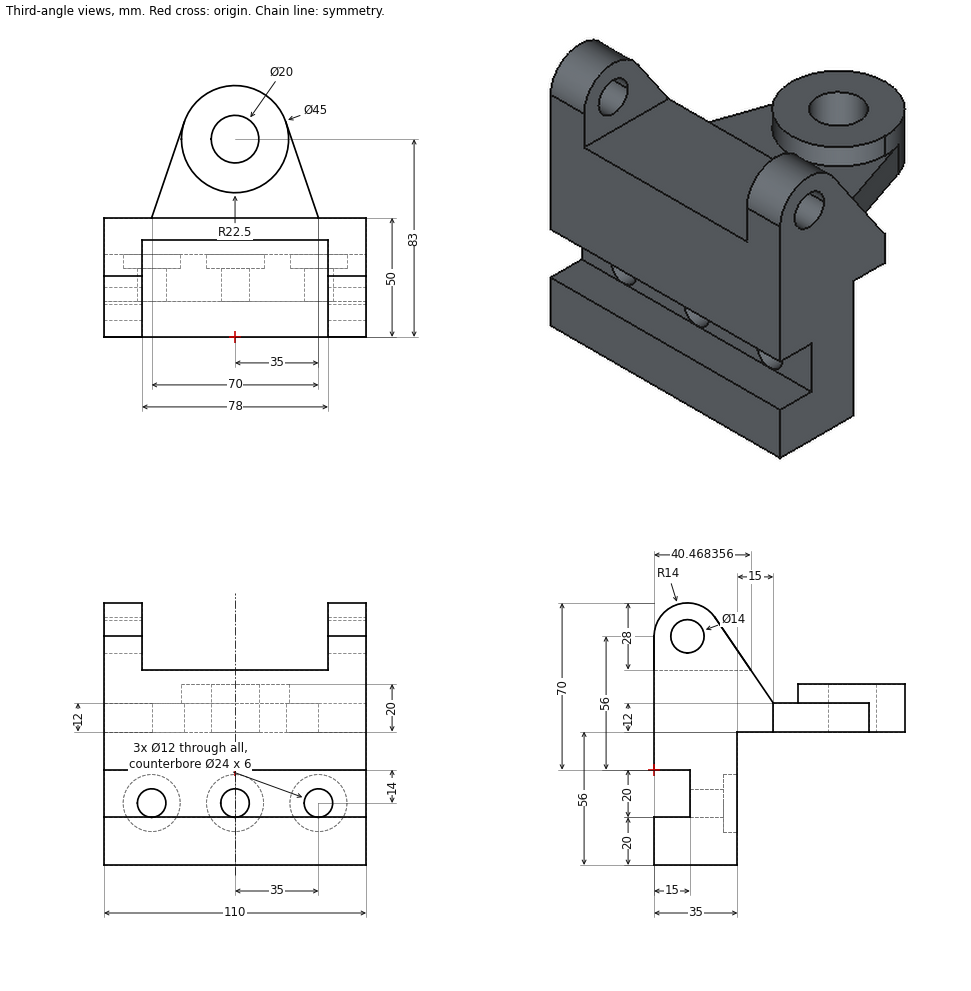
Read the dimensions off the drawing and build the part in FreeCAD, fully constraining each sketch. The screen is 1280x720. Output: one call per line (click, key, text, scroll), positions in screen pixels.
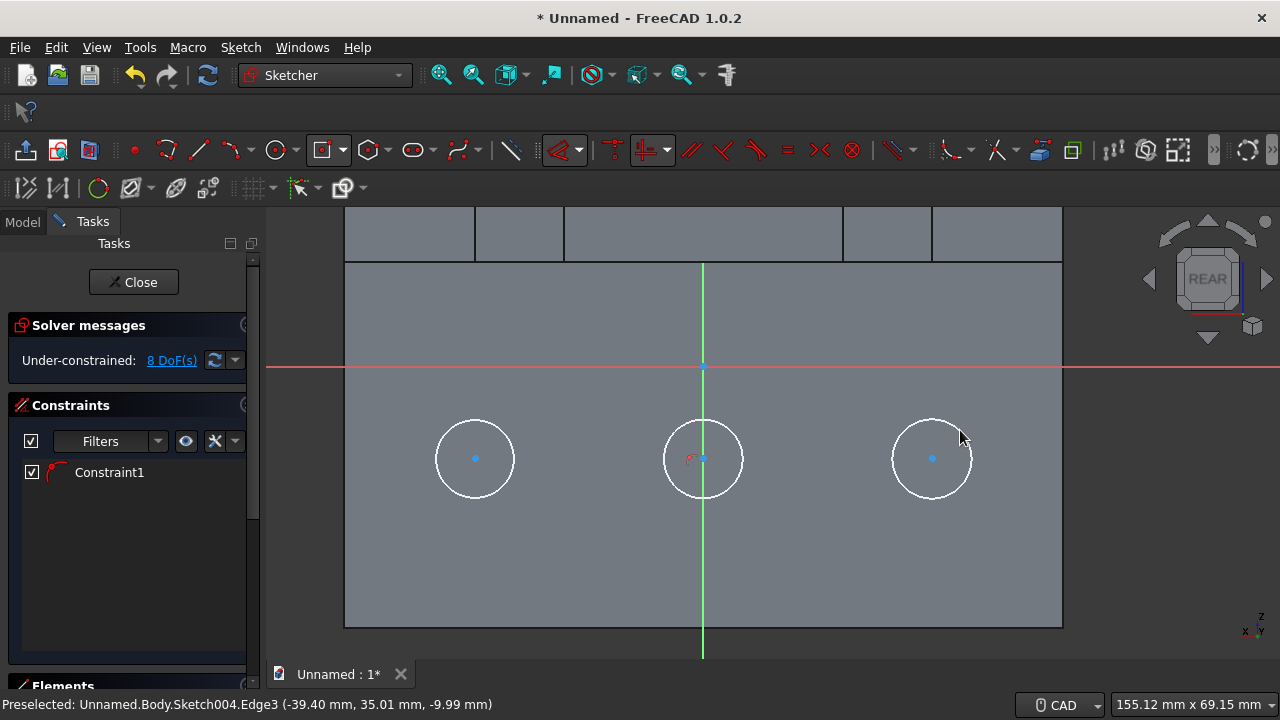
click(502, 431)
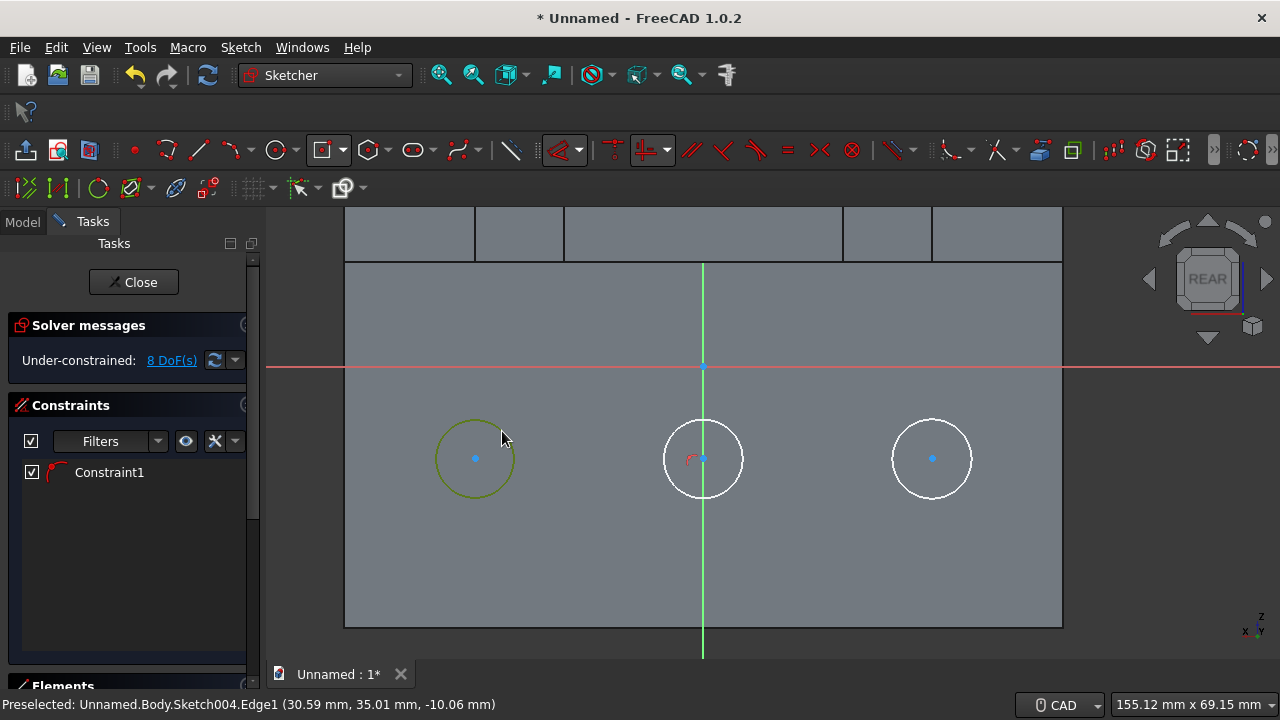
click(731, 431)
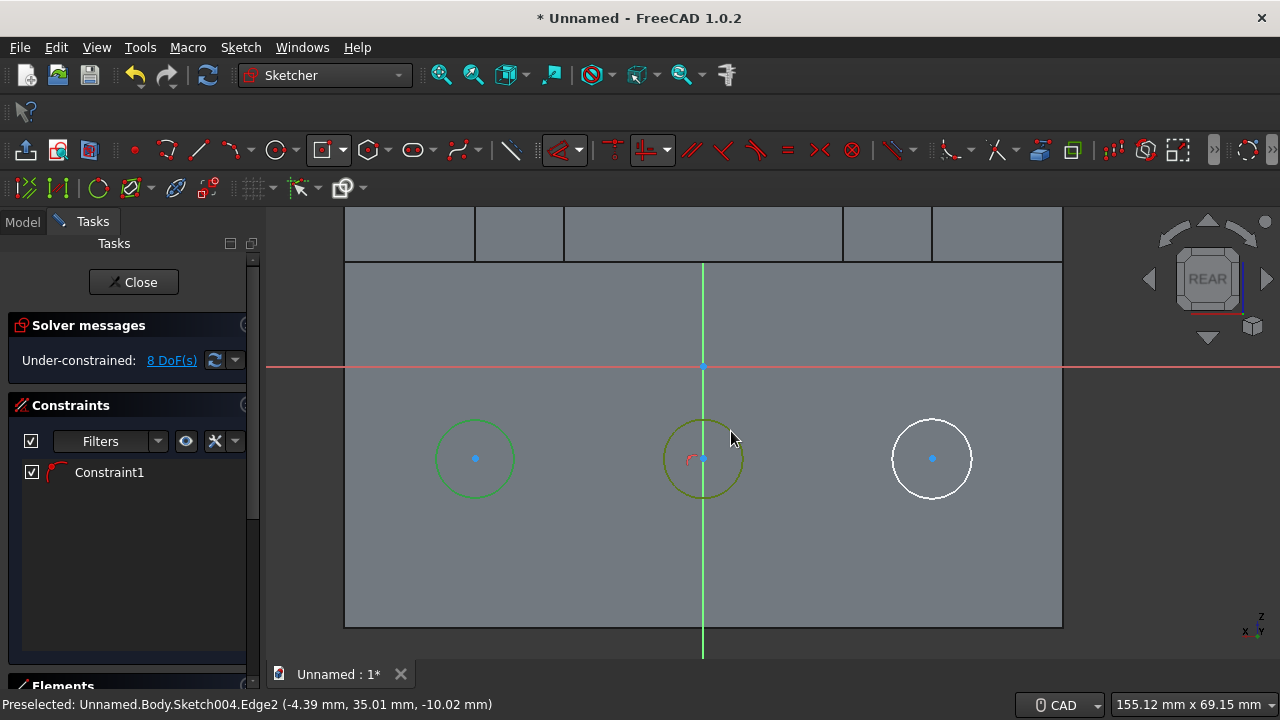
click(960, 431)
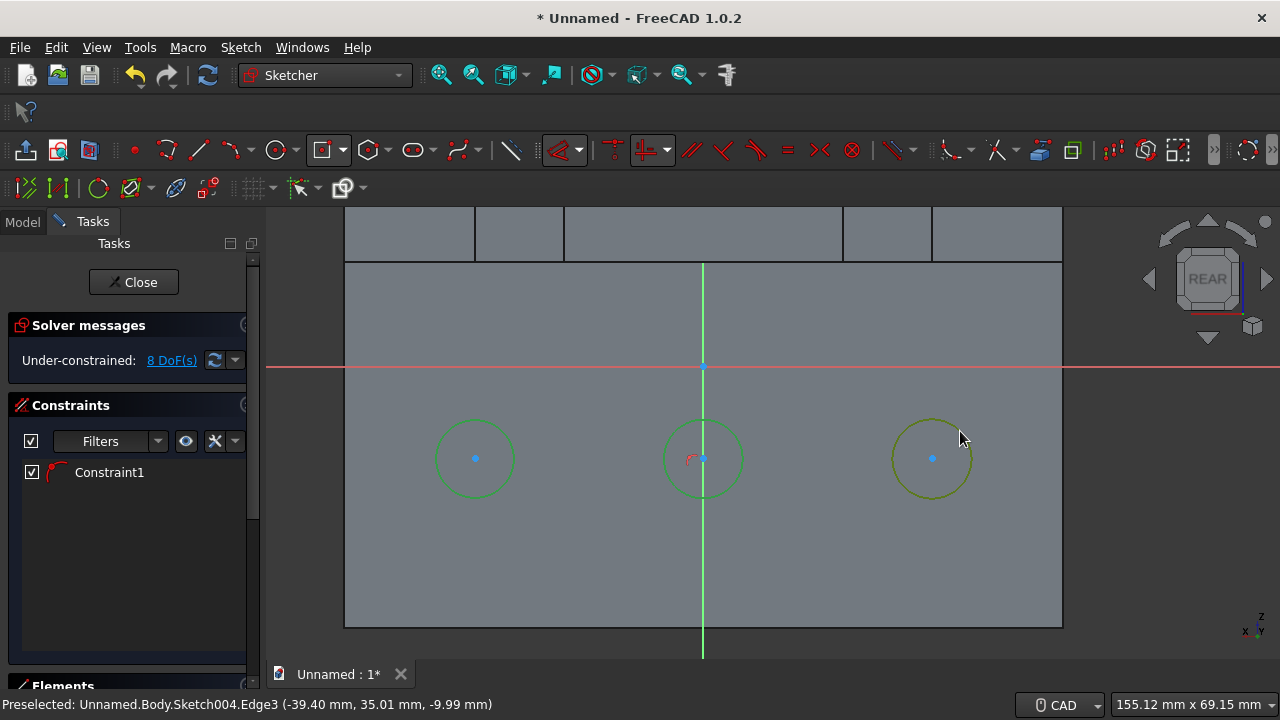
click(788, 150)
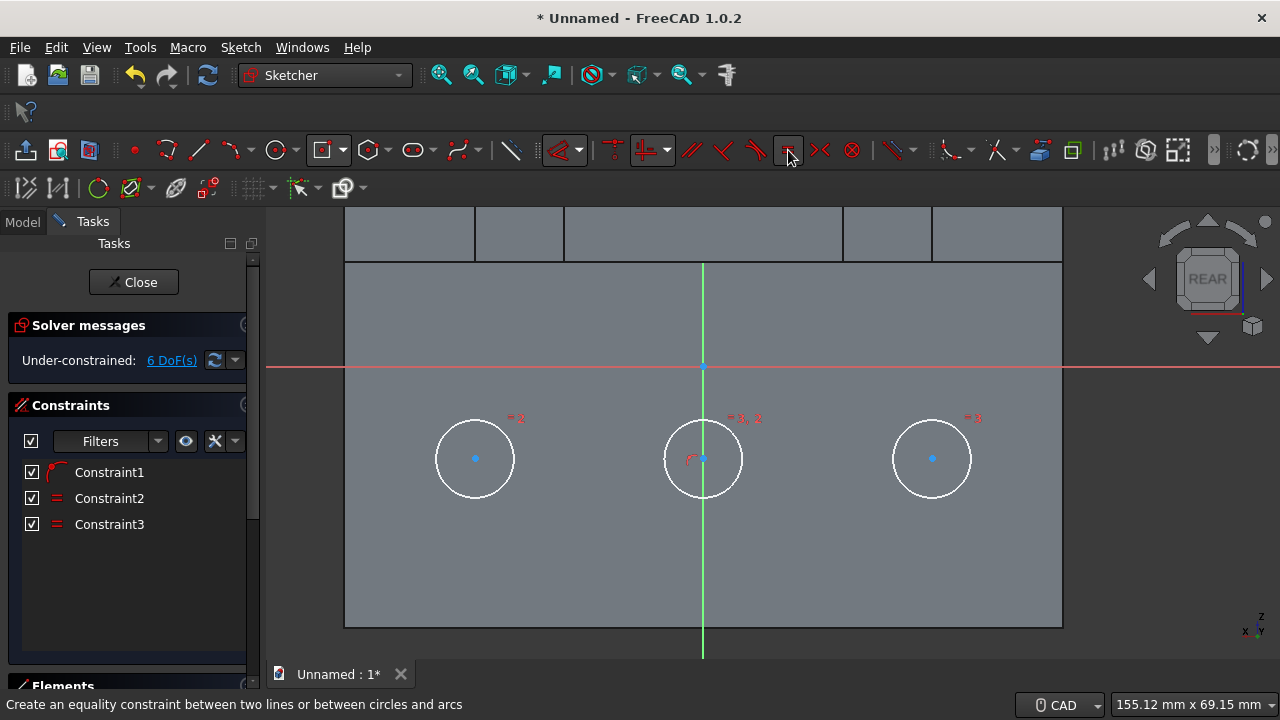
click(475, 459)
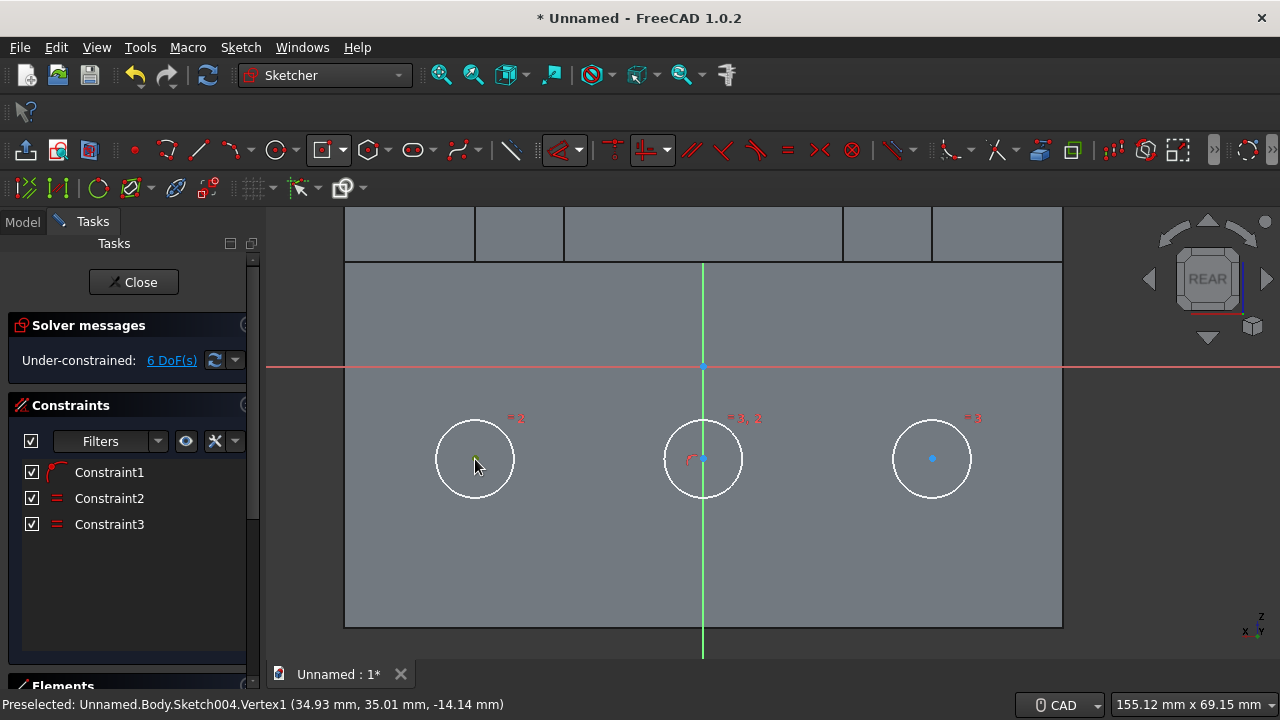
click(932, 459)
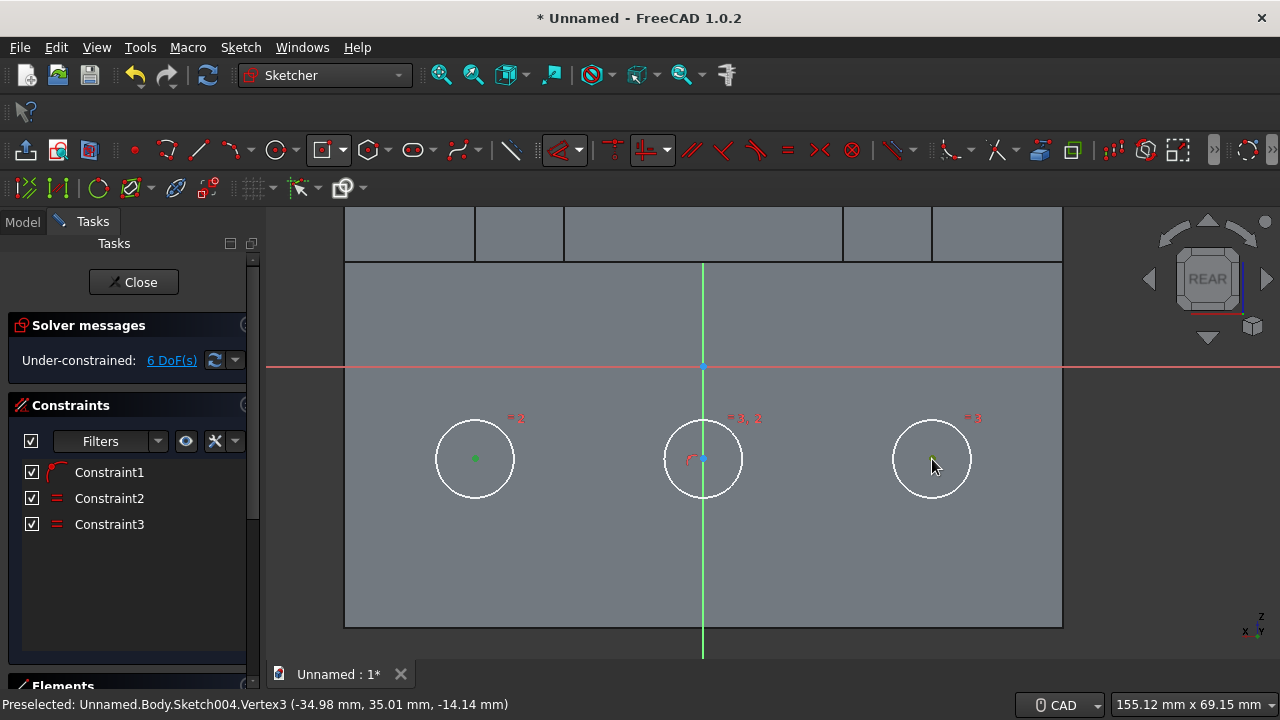
click(703, 603)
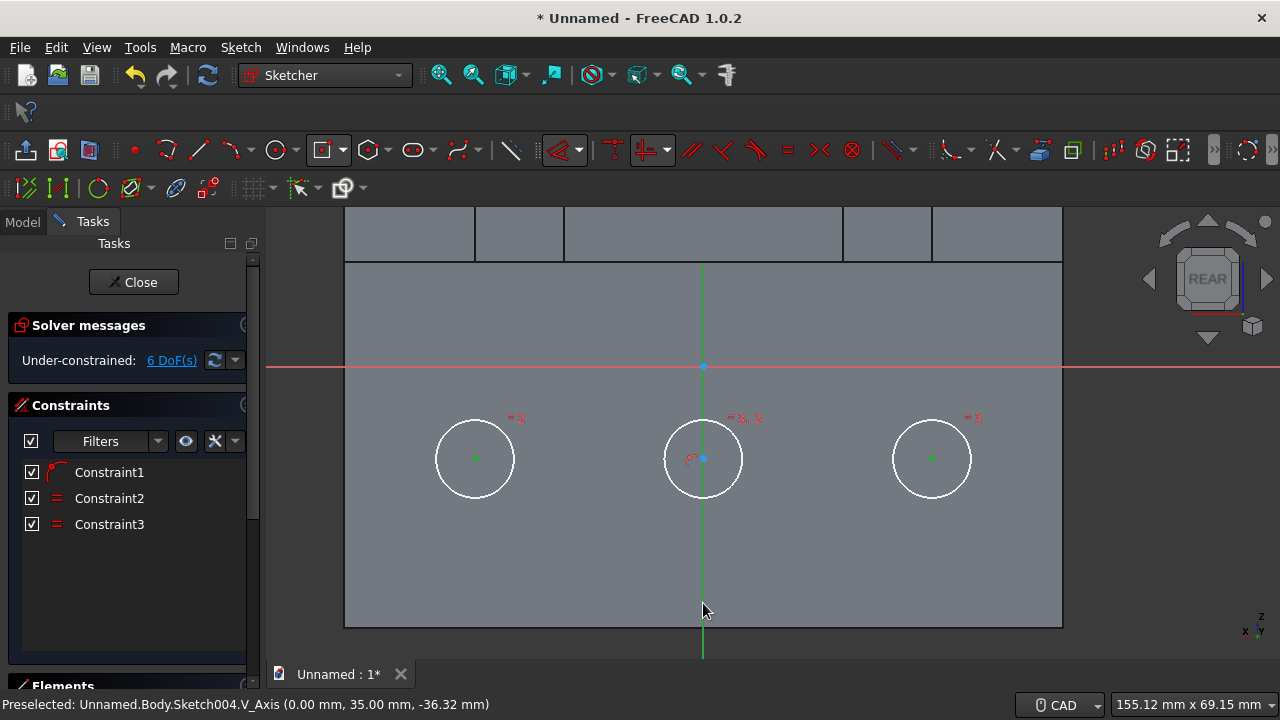
click(820, 150)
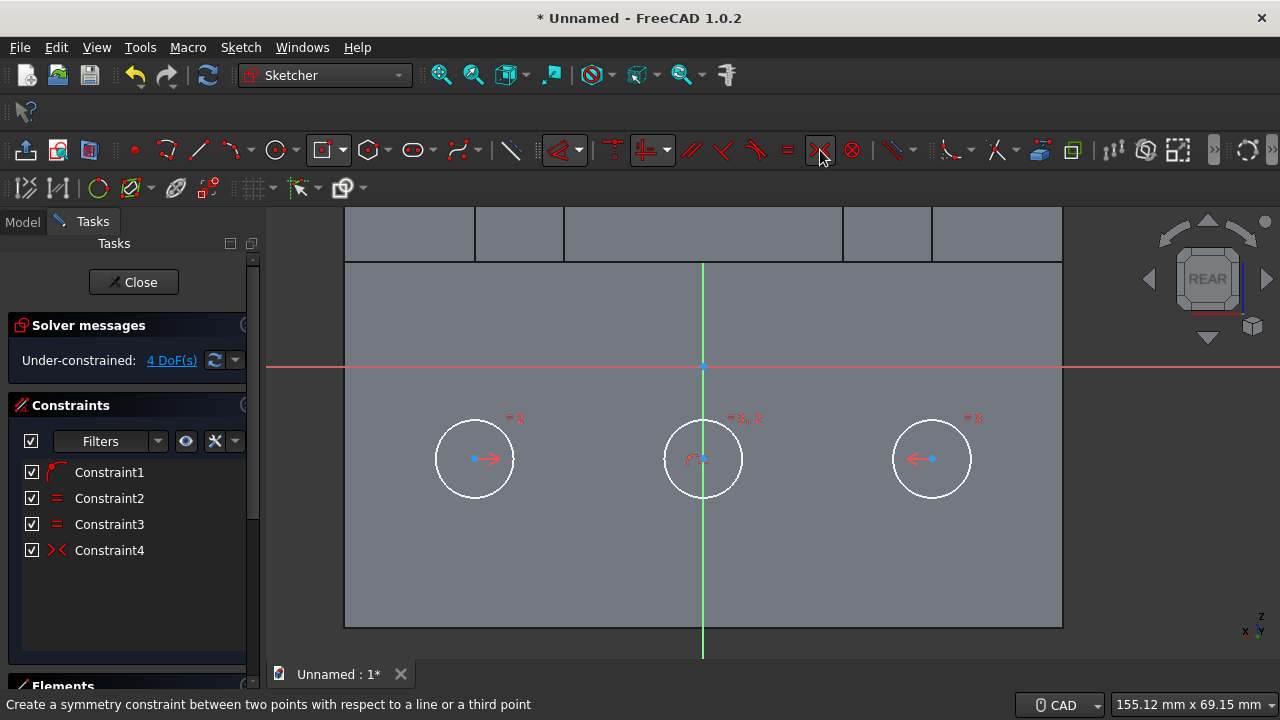
click(502, 431)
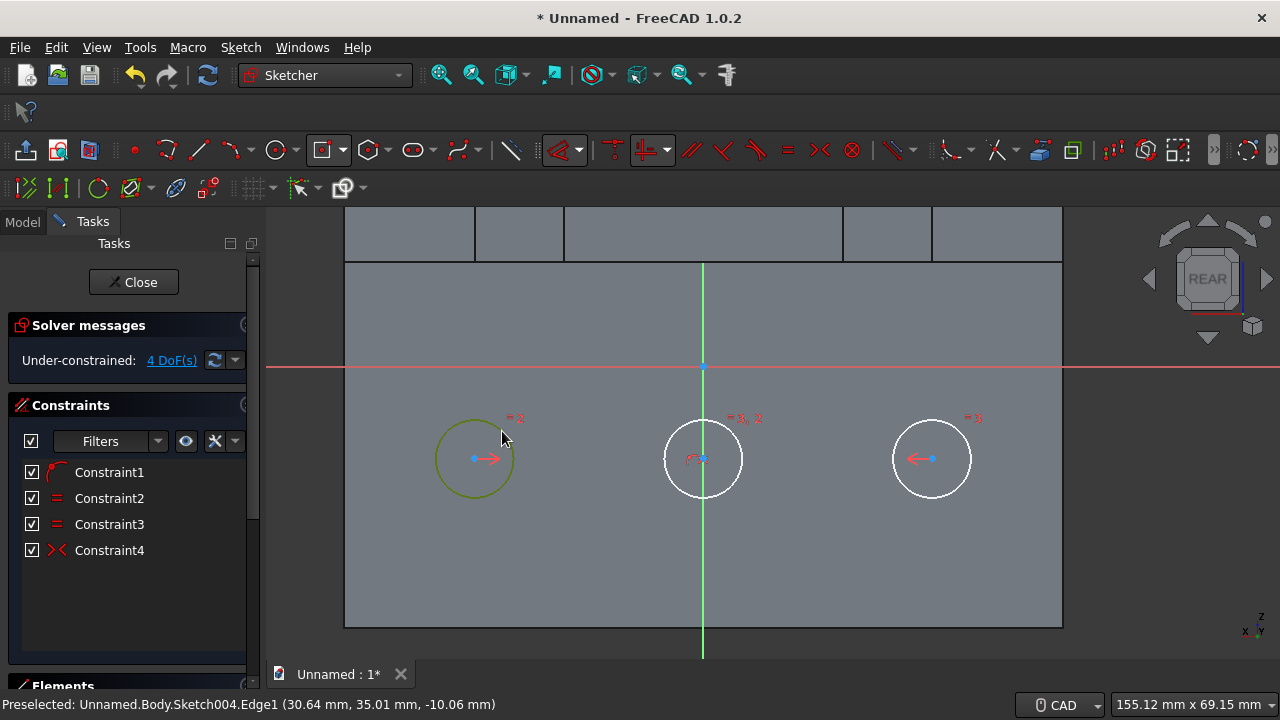
click(582, 150)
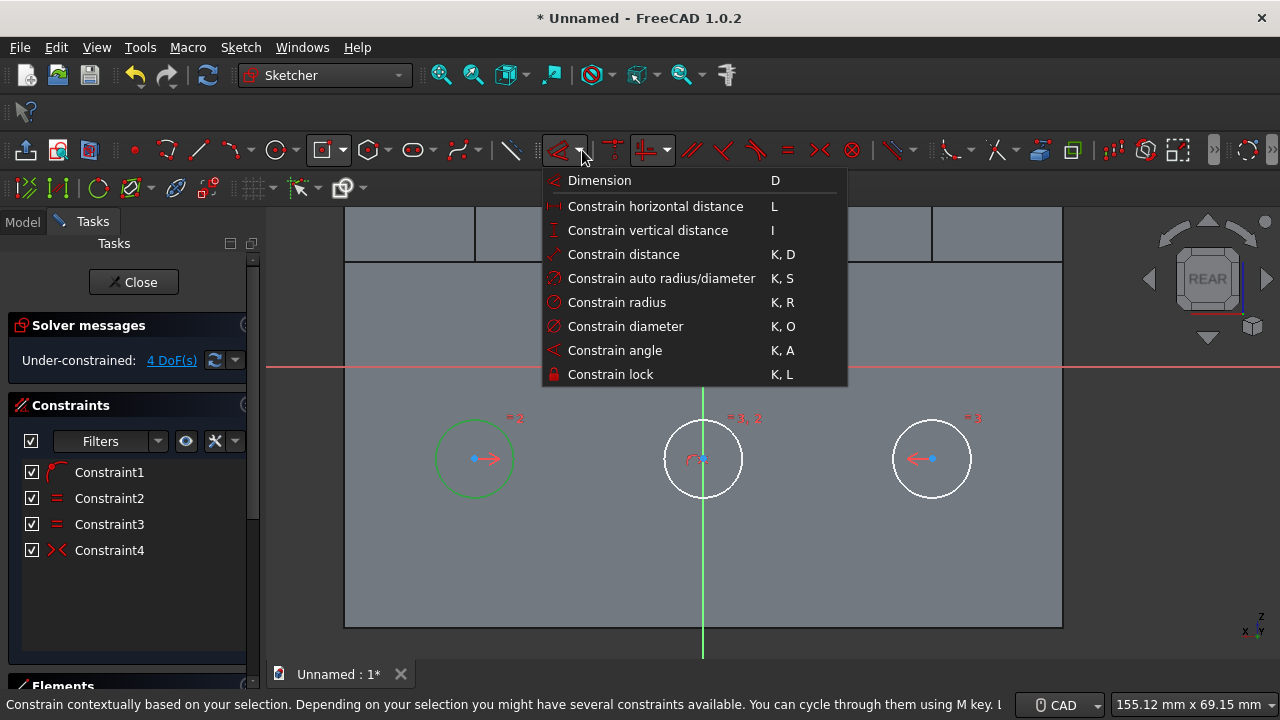
click(695, 326)